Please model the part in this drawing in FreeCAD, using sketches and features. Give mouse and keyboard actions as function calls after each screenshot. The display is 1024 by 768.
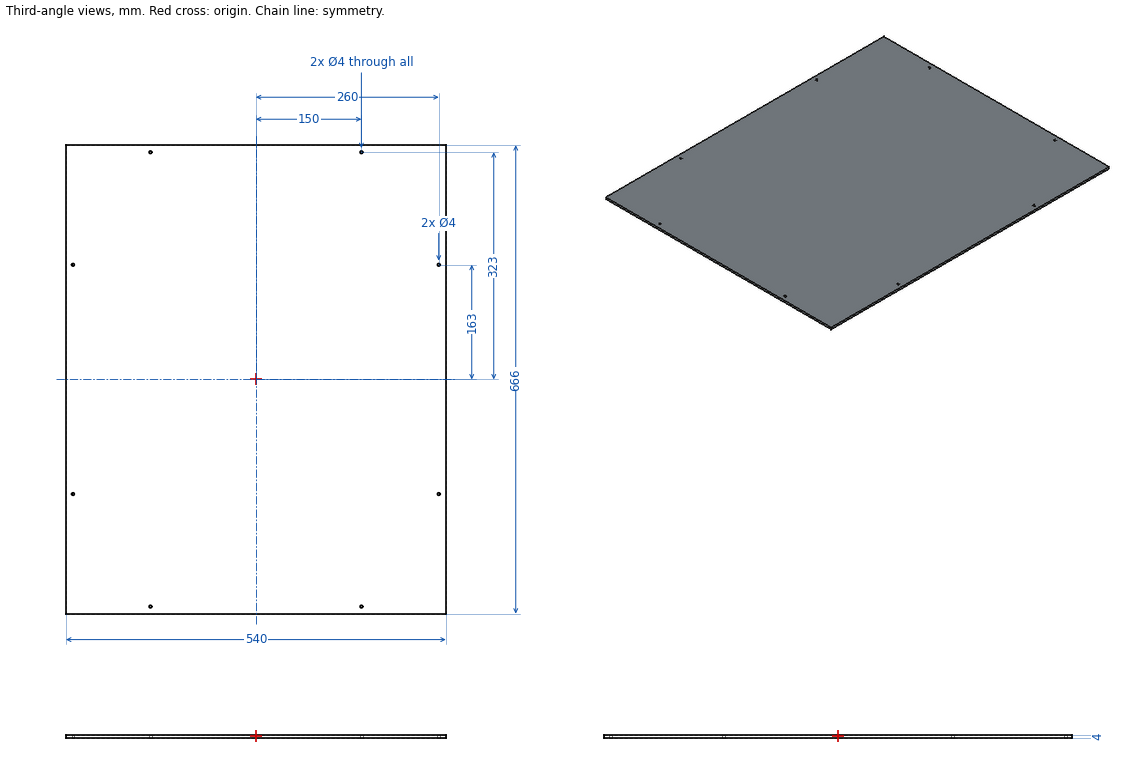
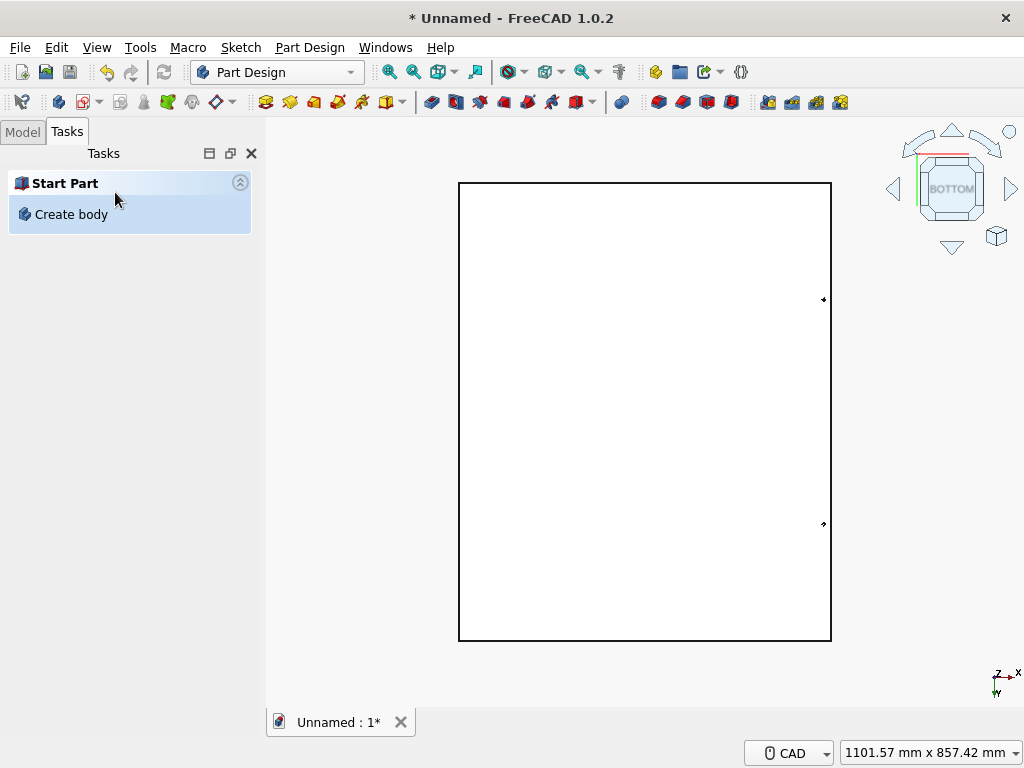
click(645, 411)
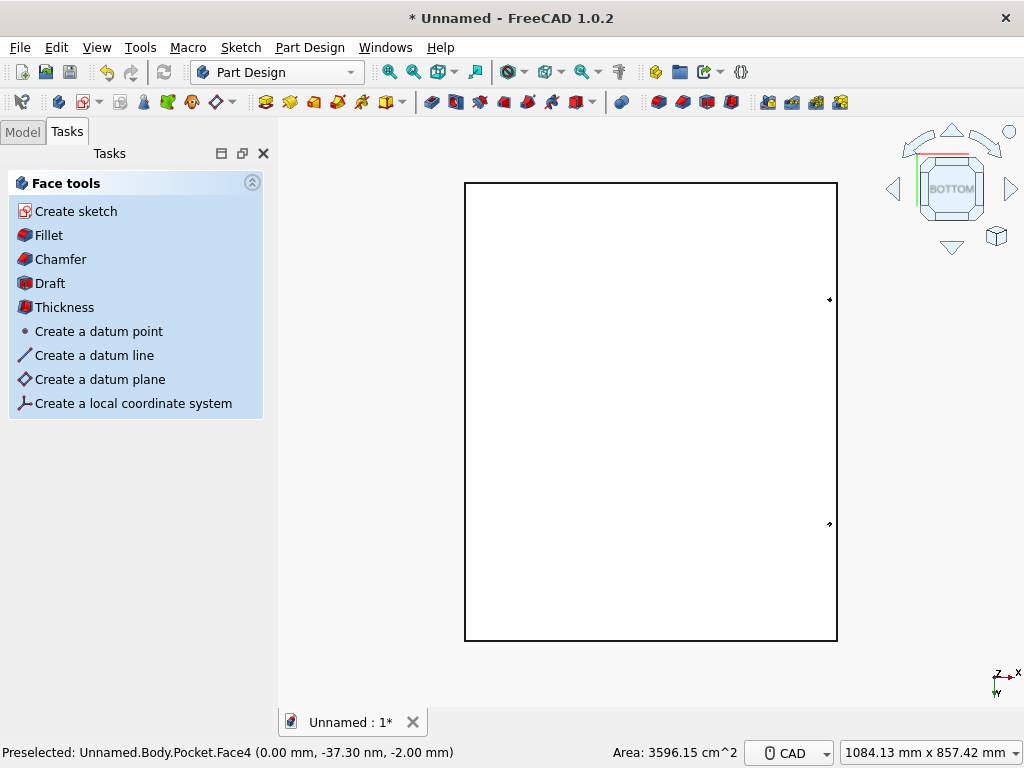
click(84, 102)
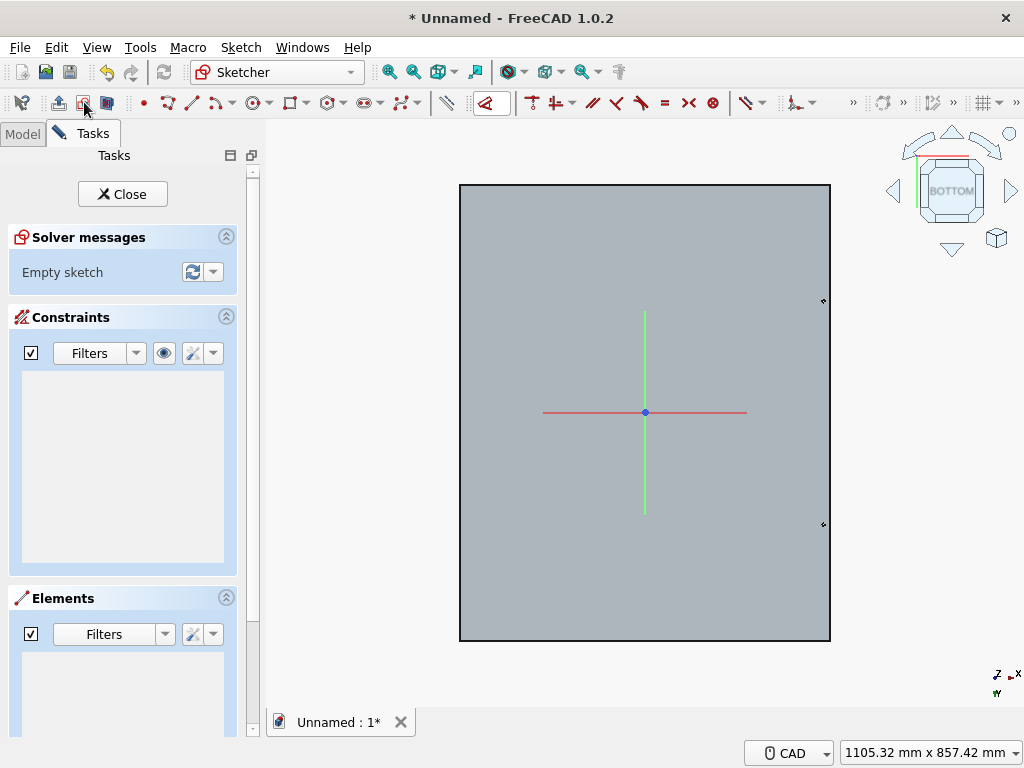
scroll(728, 660, up, 3)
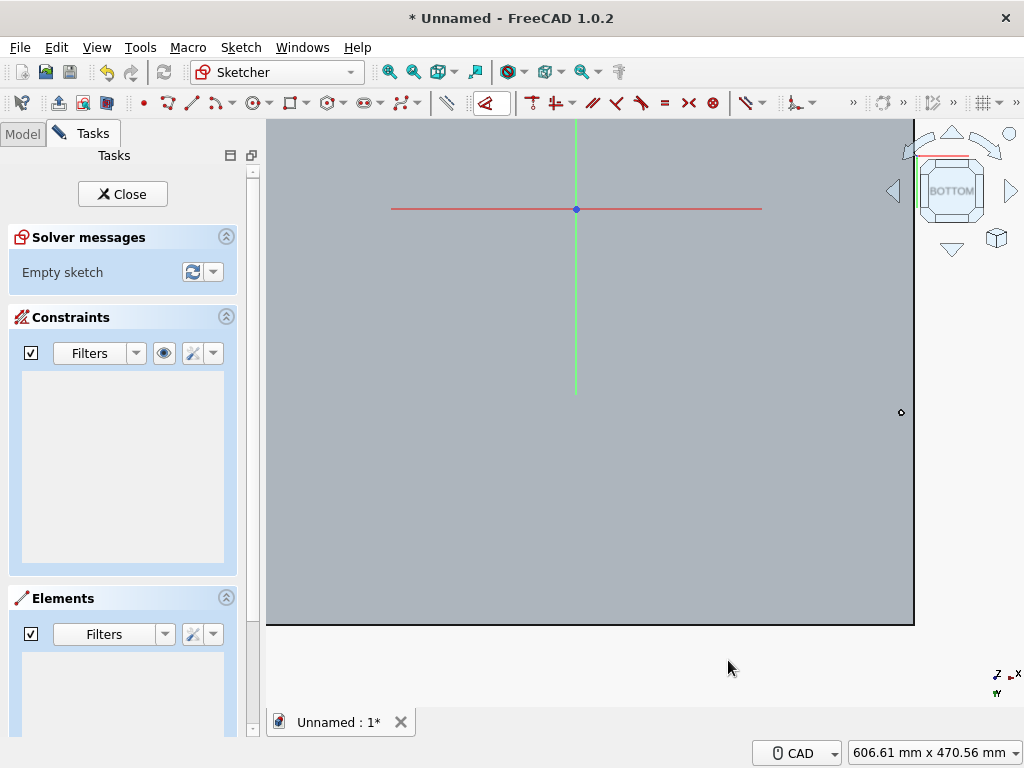
click(254, 104)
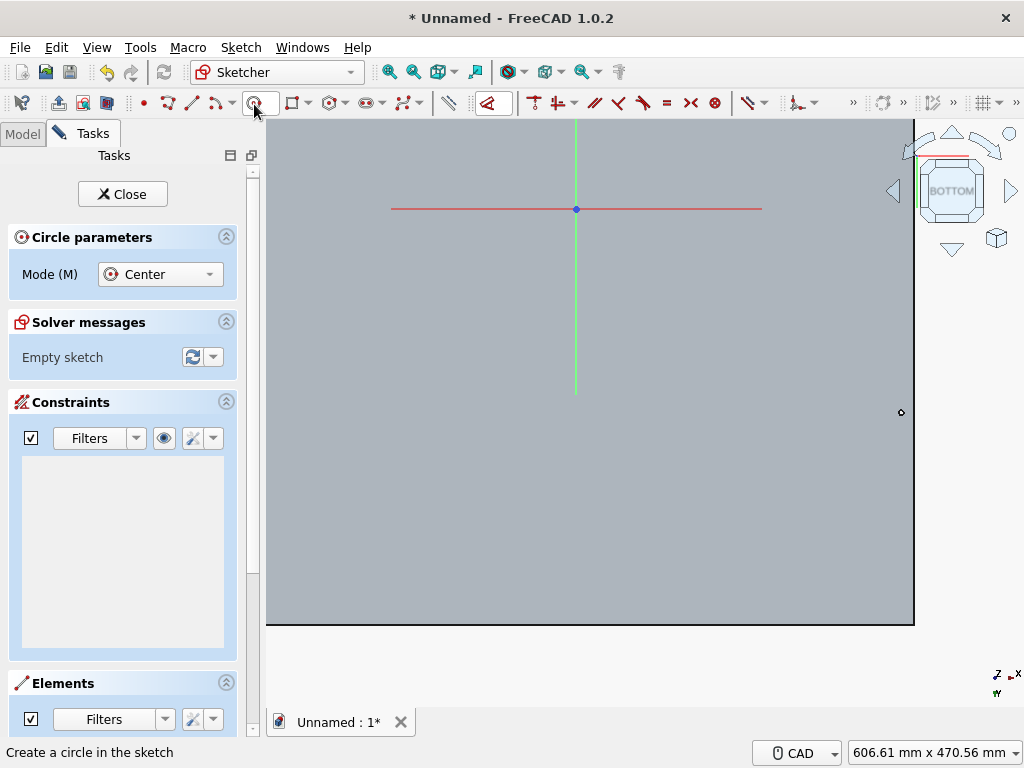
scroll(764, 613, up, 12)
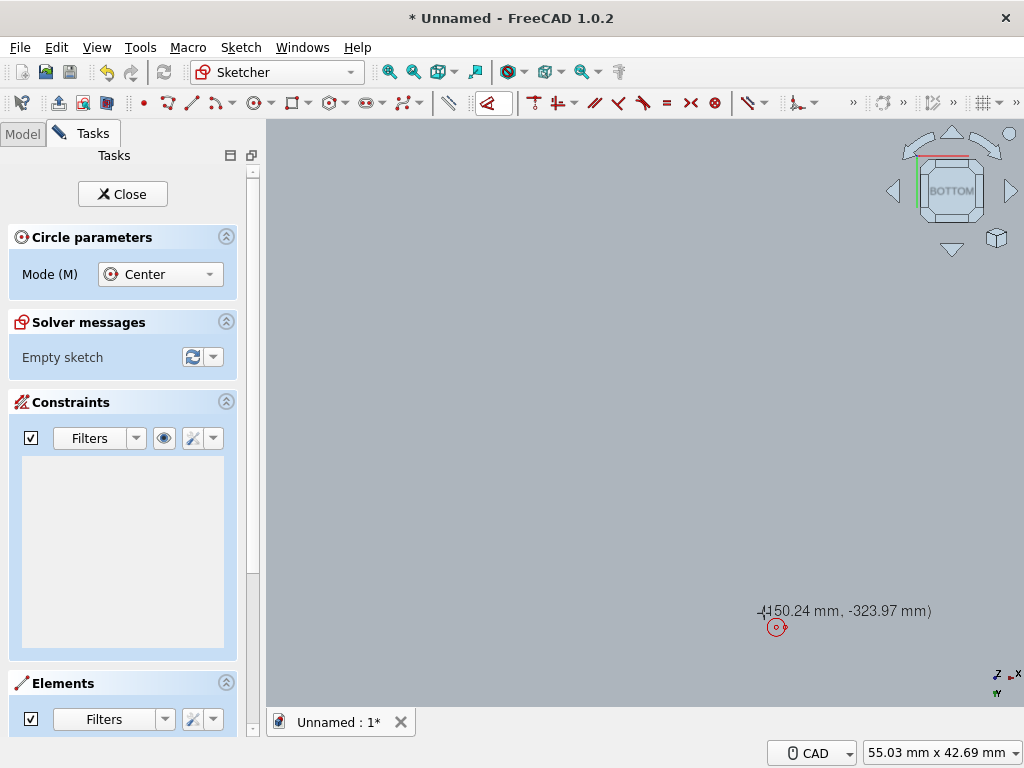
scroll(765, 615, down, 12)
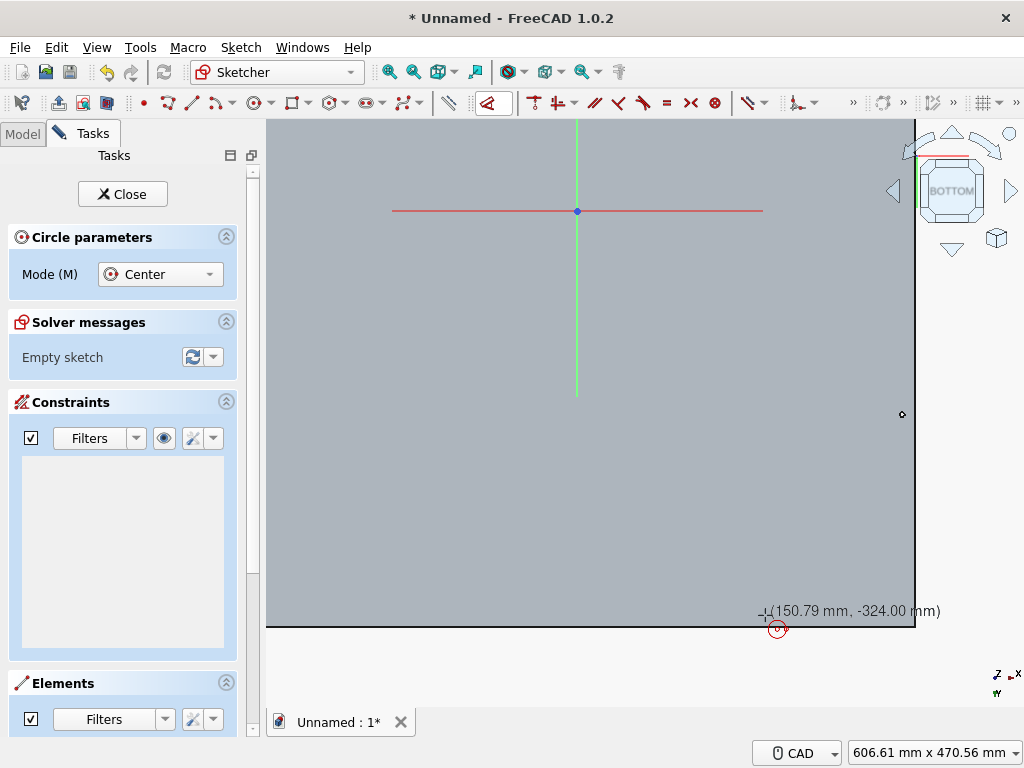
click(765, 615)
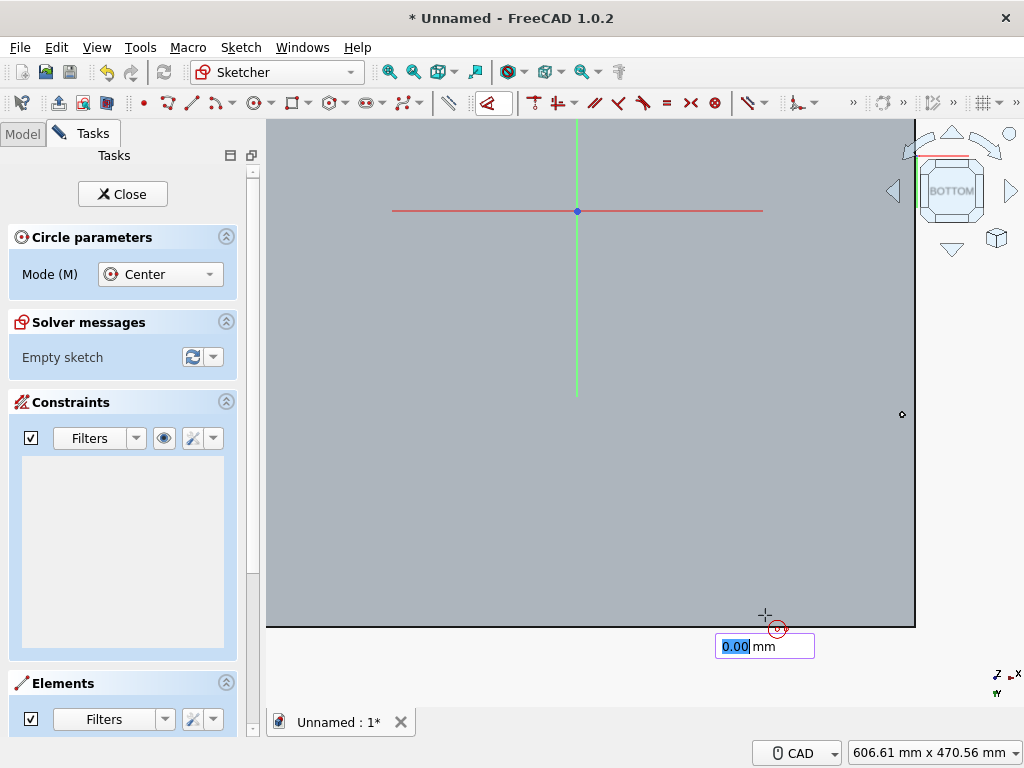
scroll(766, 613, up, 10)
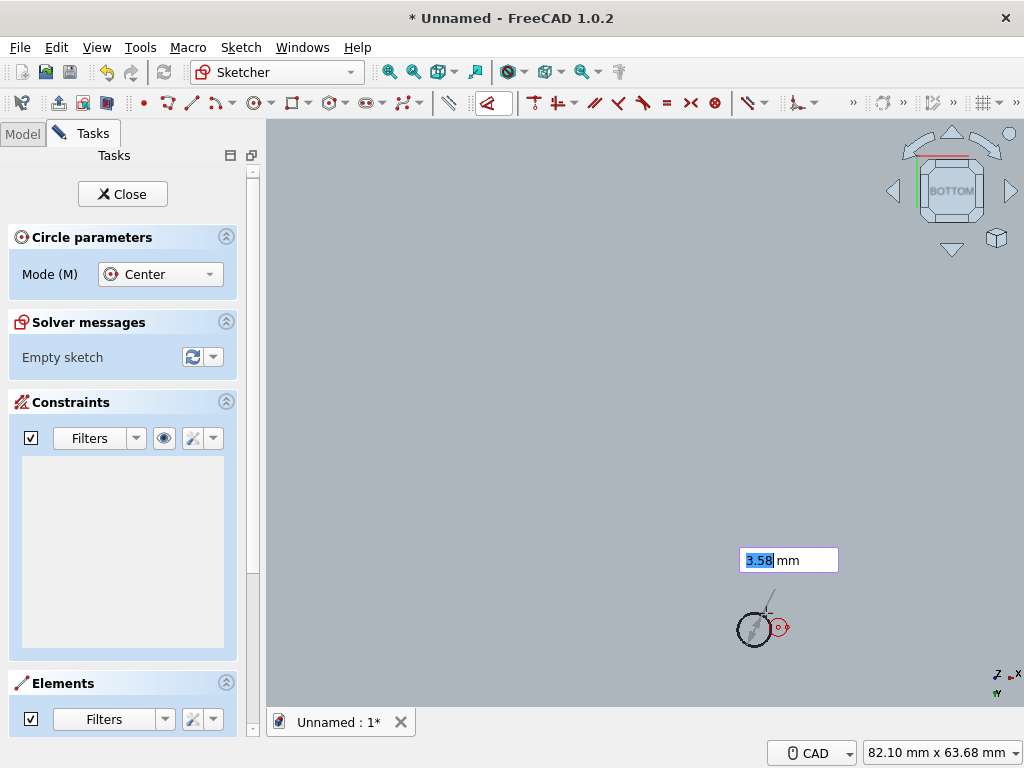
click(765, 606)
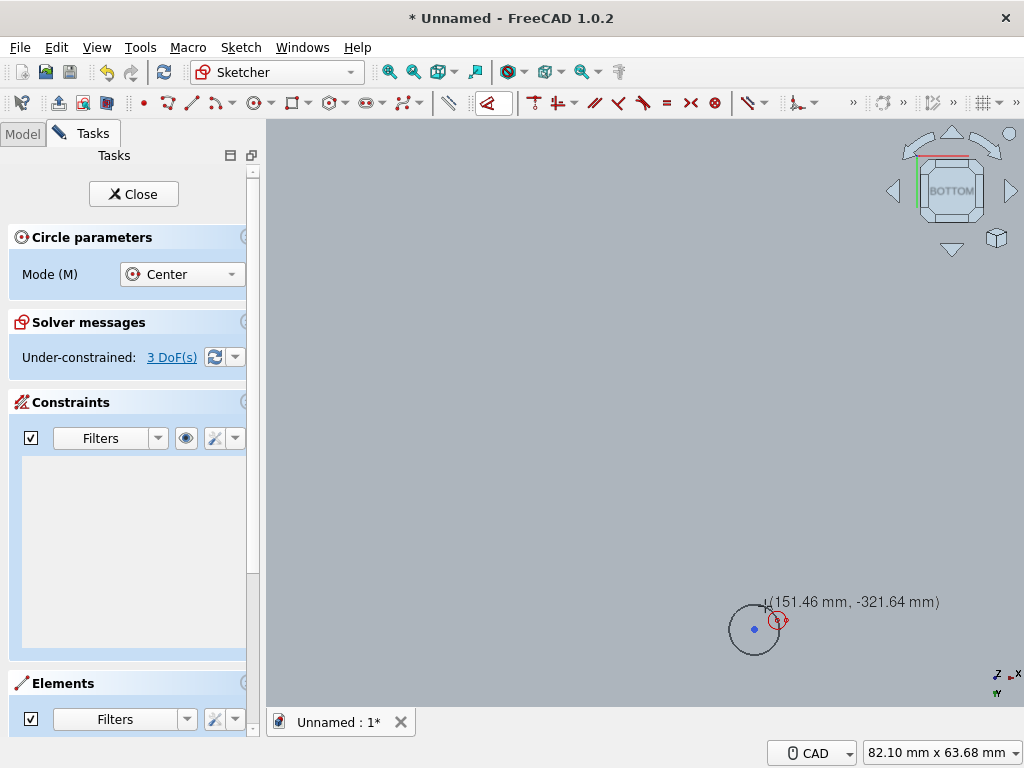
scroll(766, 613, down, 10)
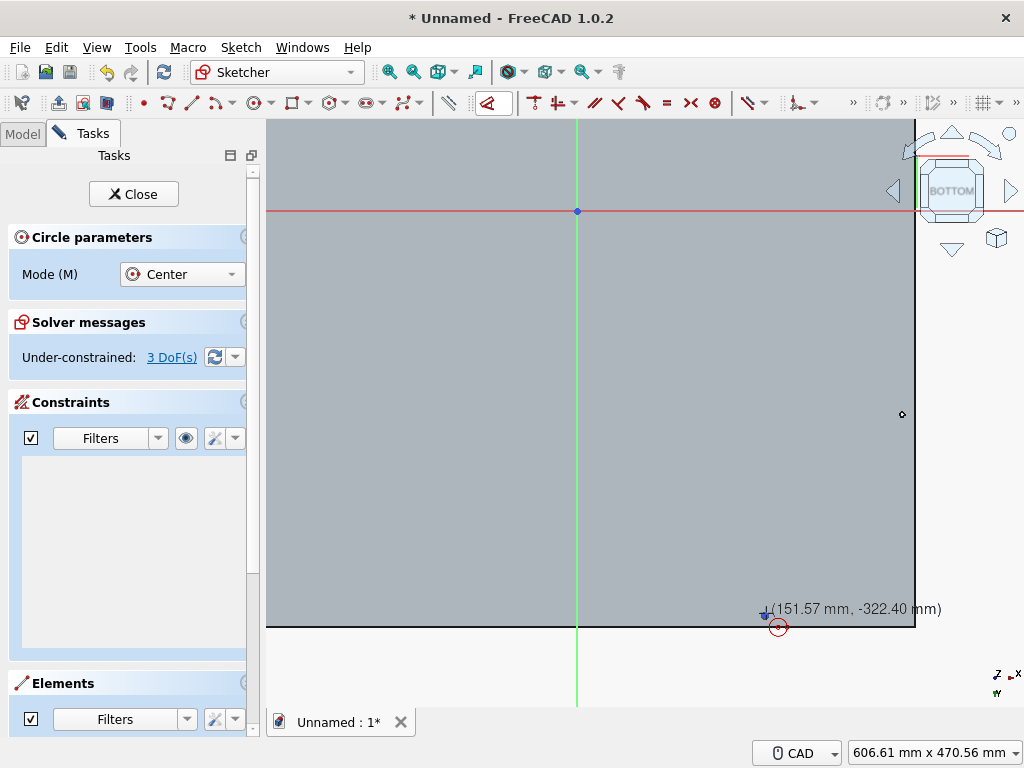
scroll(390, 615, up, 12)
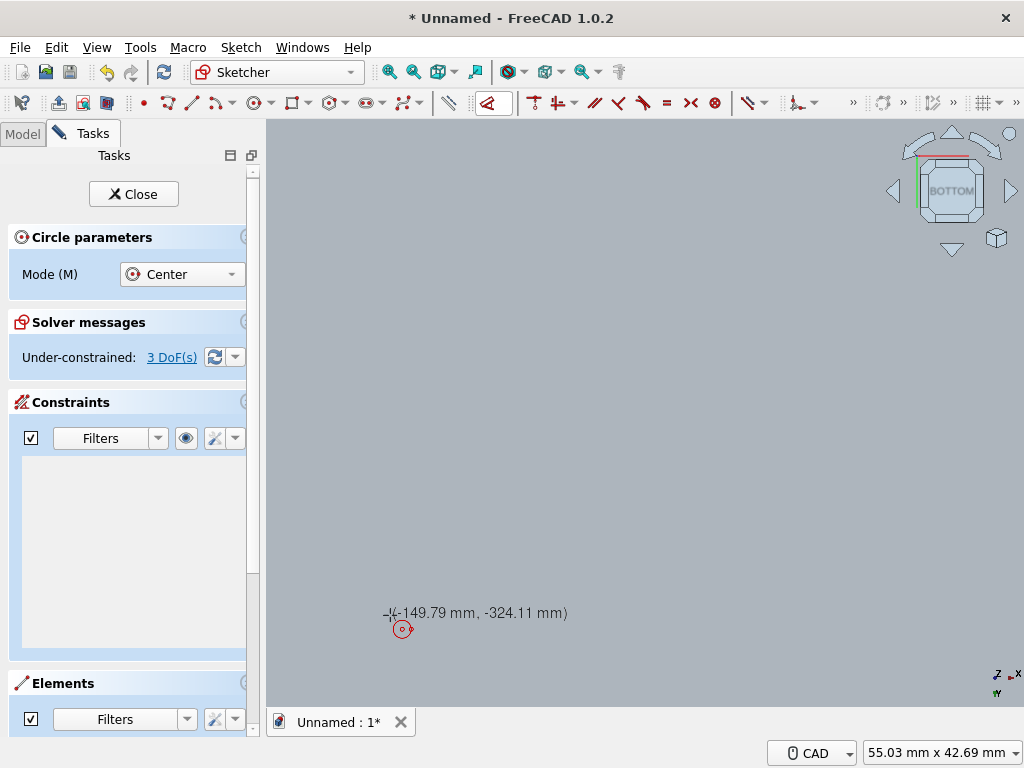
scroll(389, 615, down, 12)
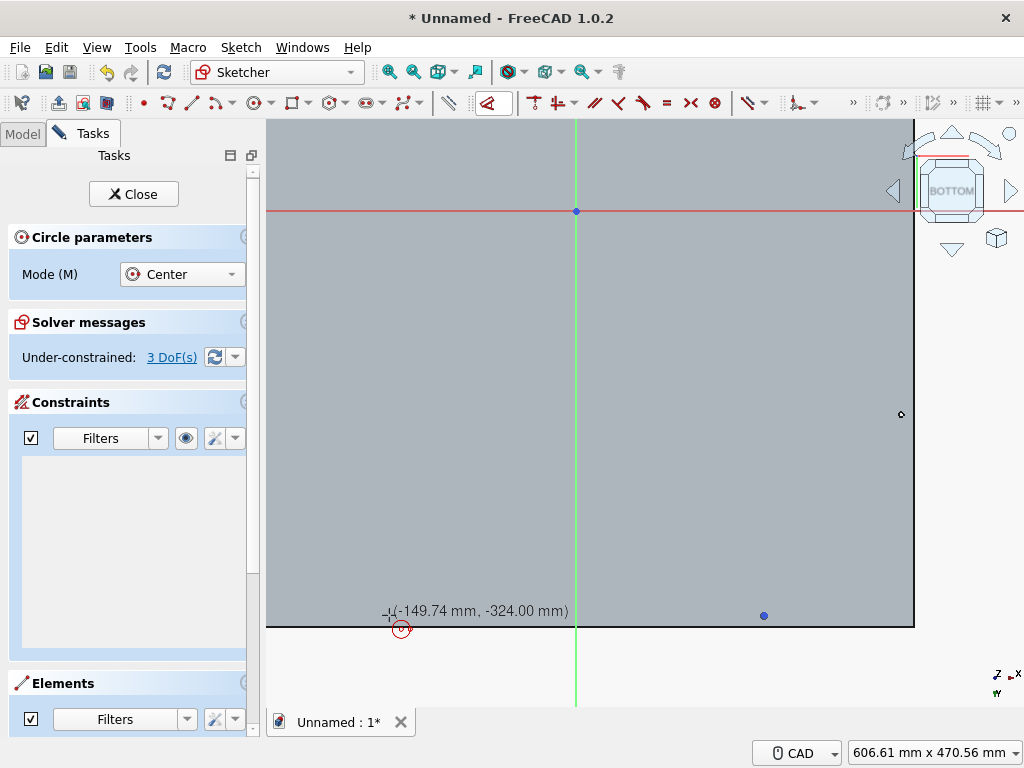
click(389, 615)